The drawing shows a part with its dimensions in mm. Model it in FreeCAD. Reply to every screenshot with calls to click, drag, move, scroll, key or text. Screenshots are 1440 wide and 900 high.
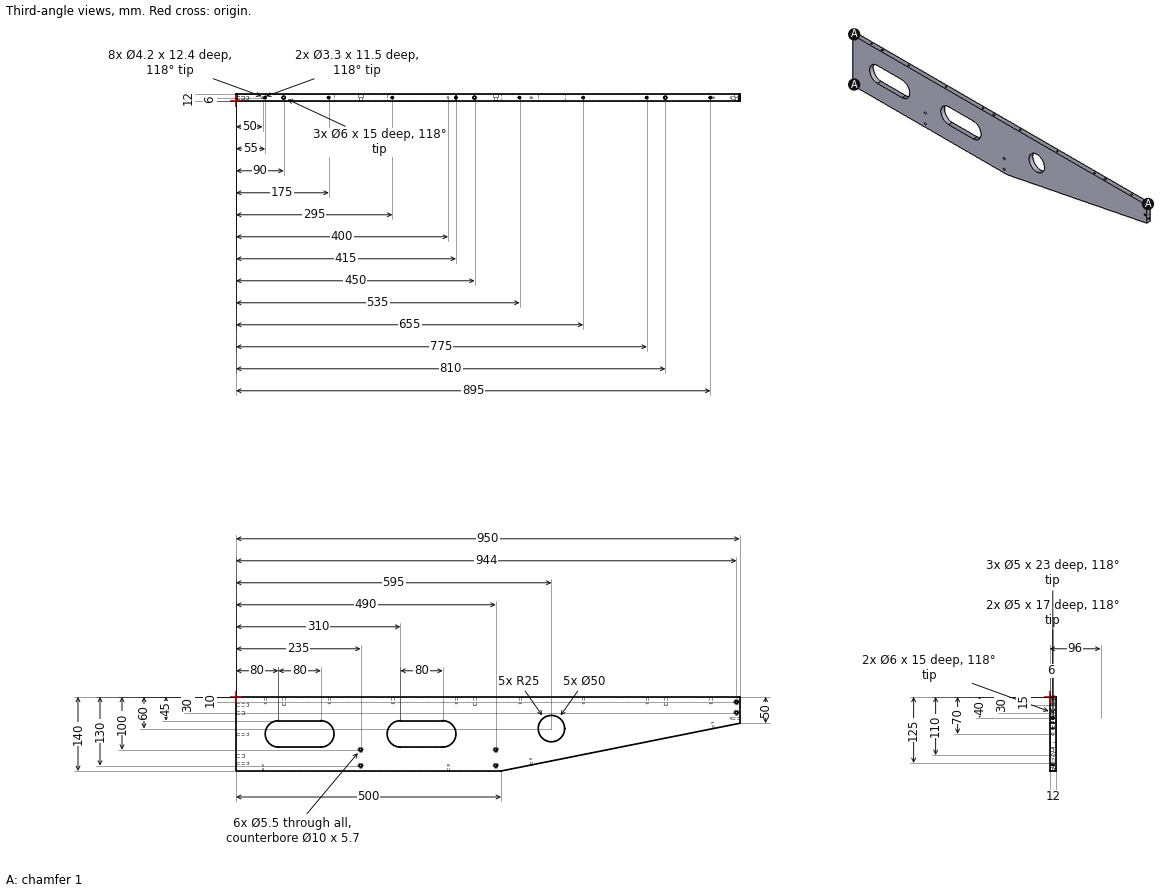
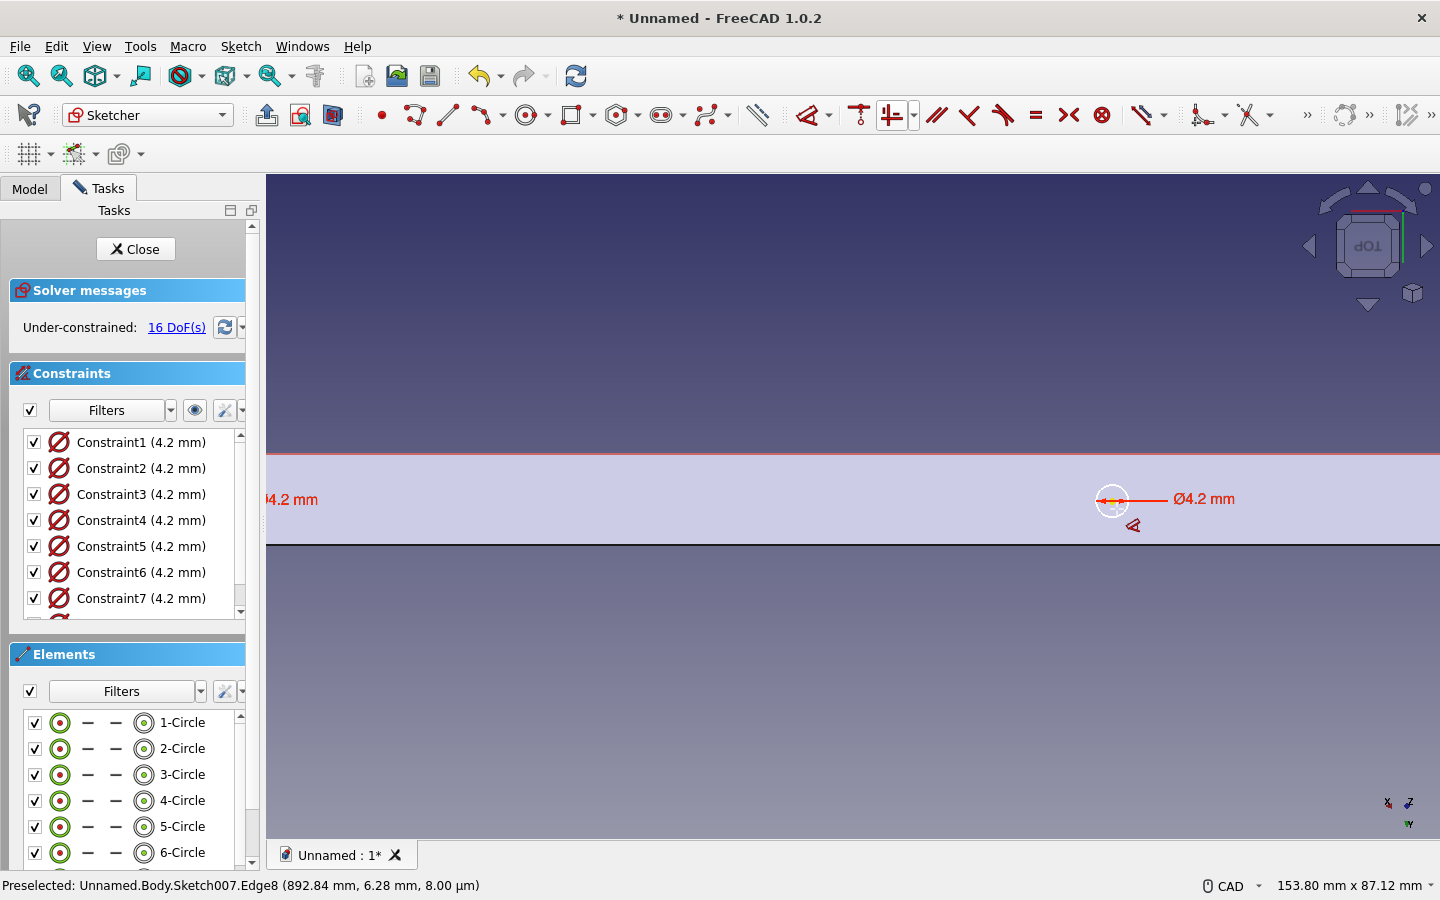
click(1112, 501)
click(1078, 478)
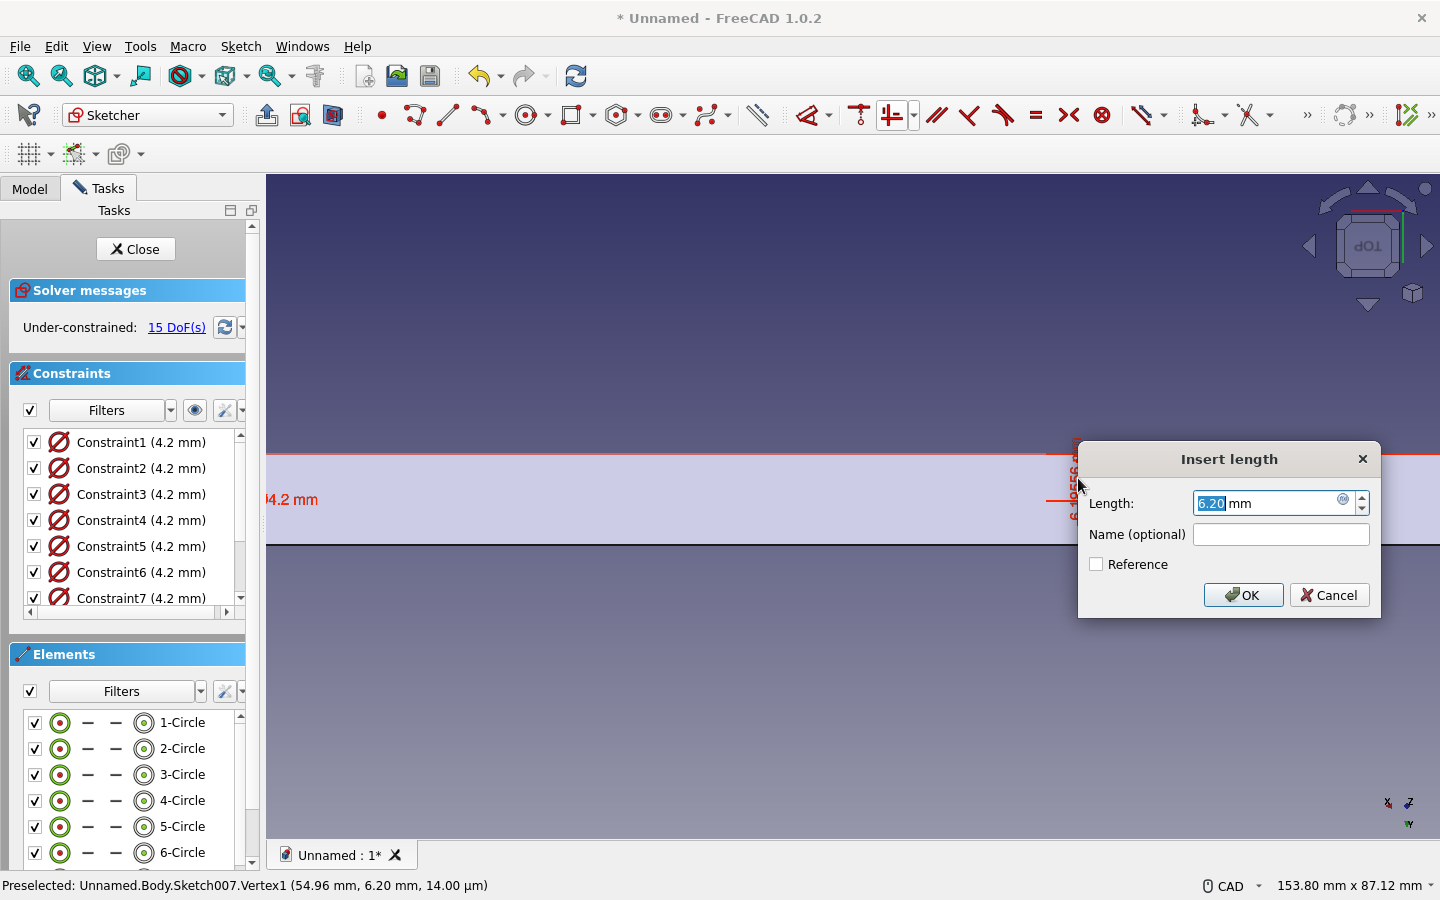
text(6)
key(Return)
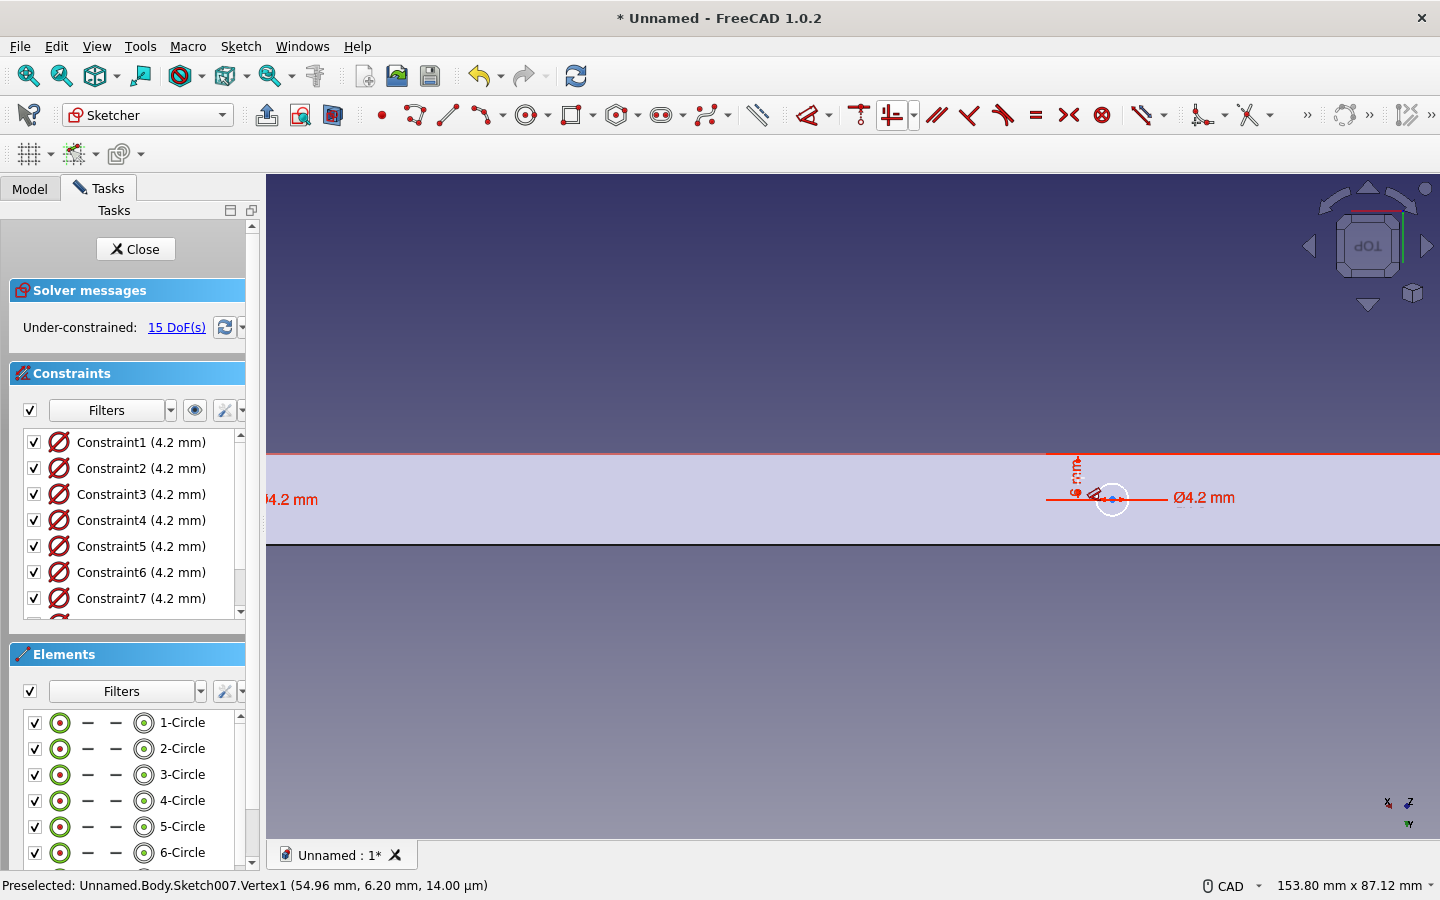
scroll(1118, 509, down, 11)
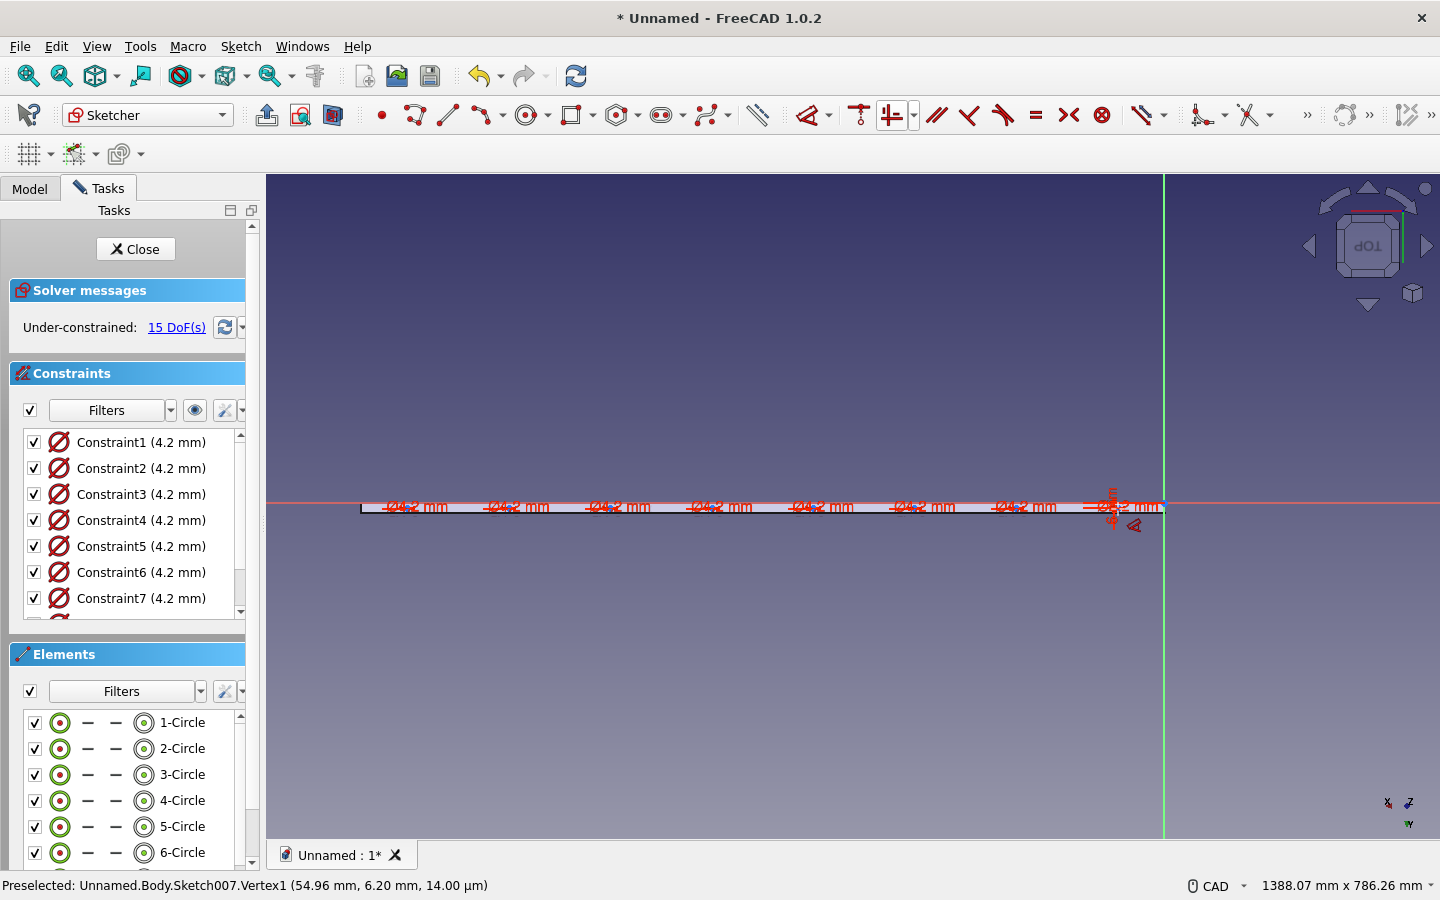
scroll(1016, 509, up, 11)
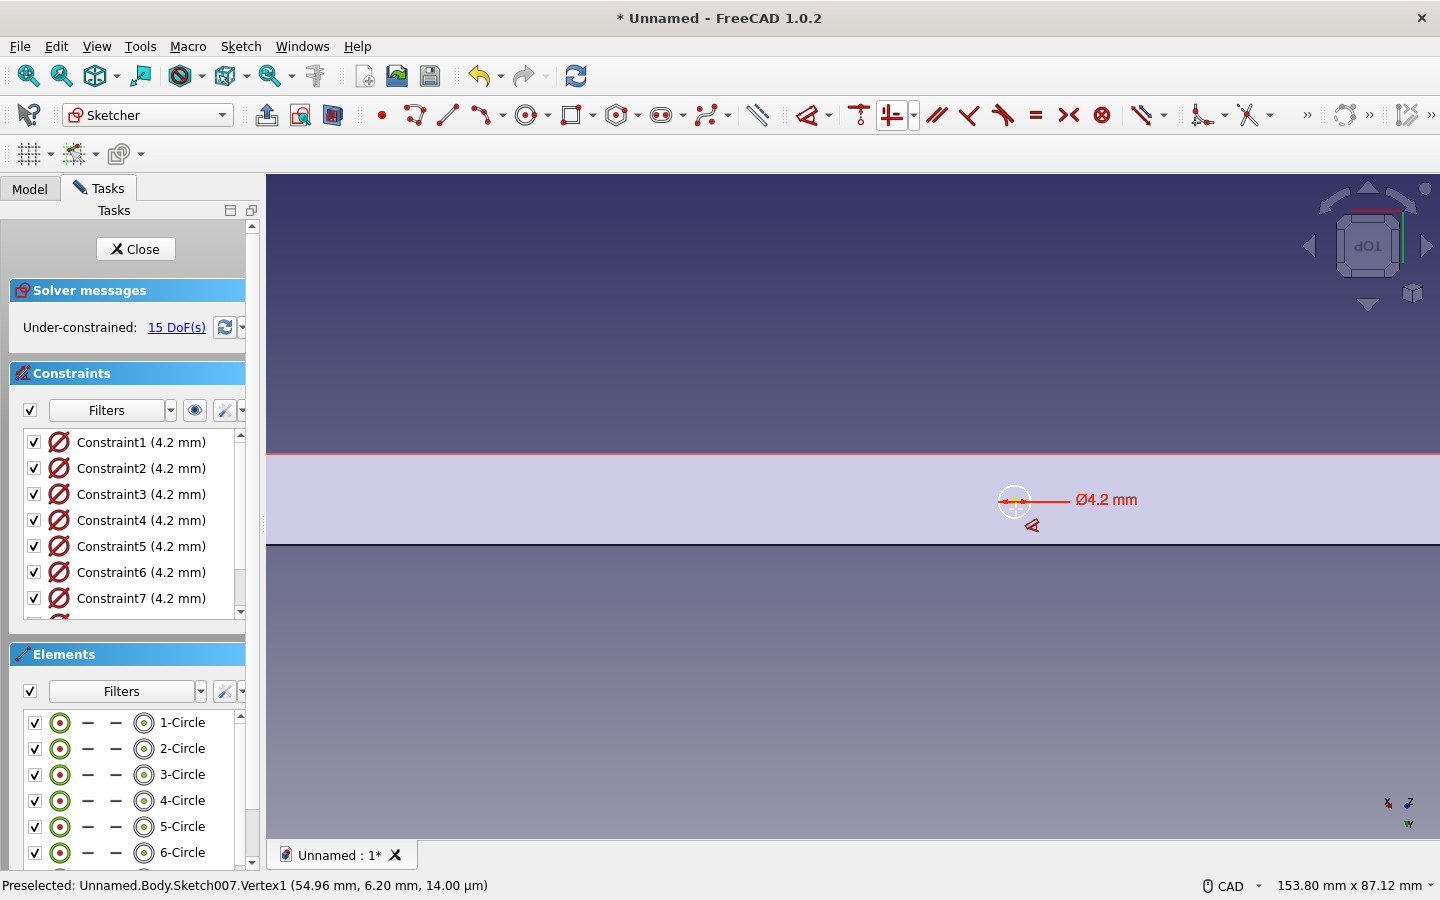
click(1015, 502)
click(981, 478)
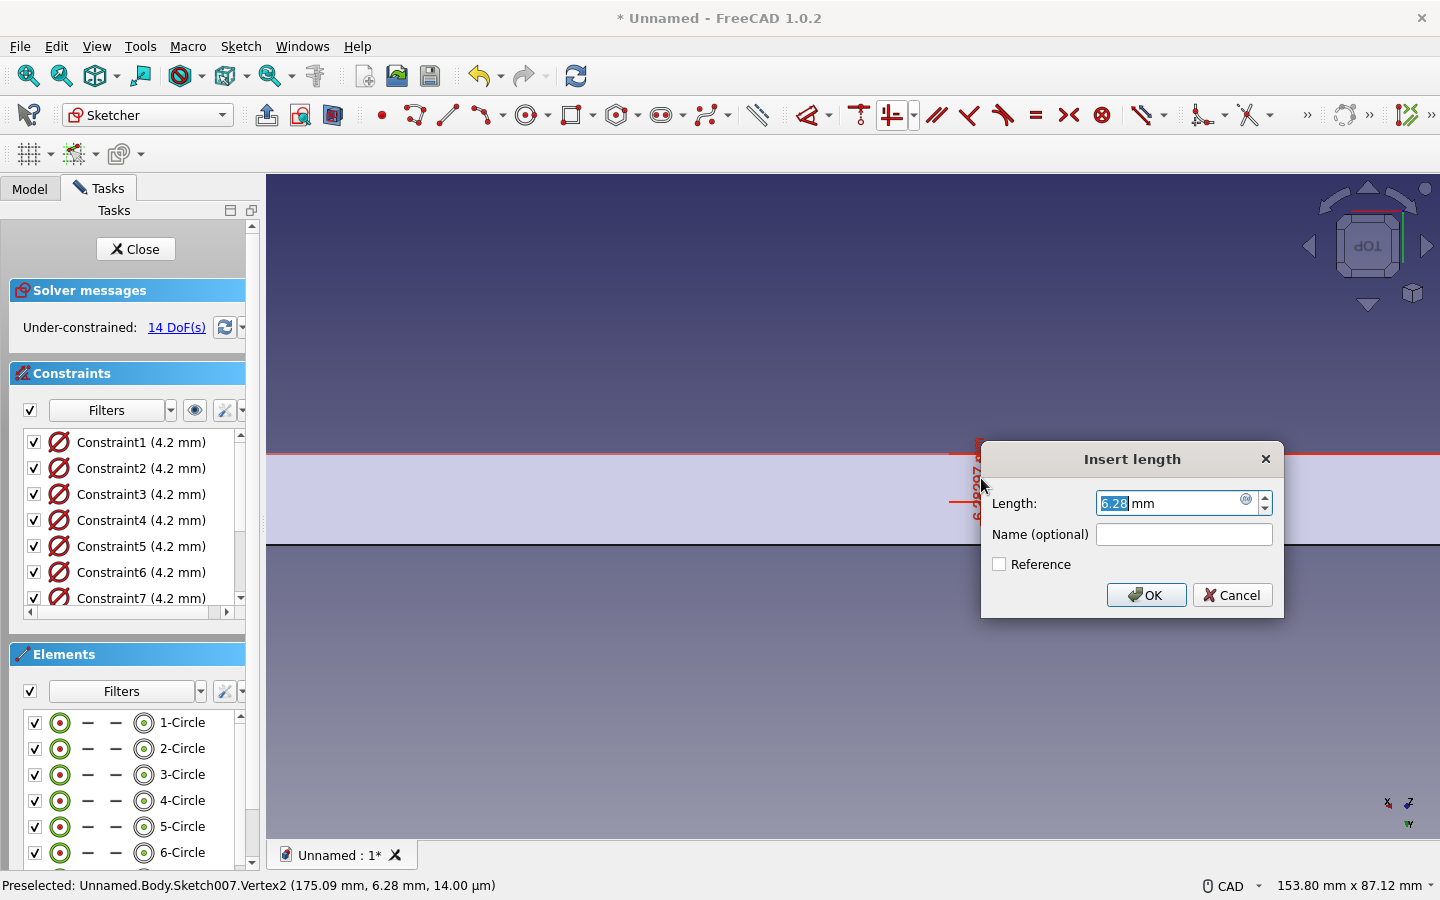
text(6)
key(Return)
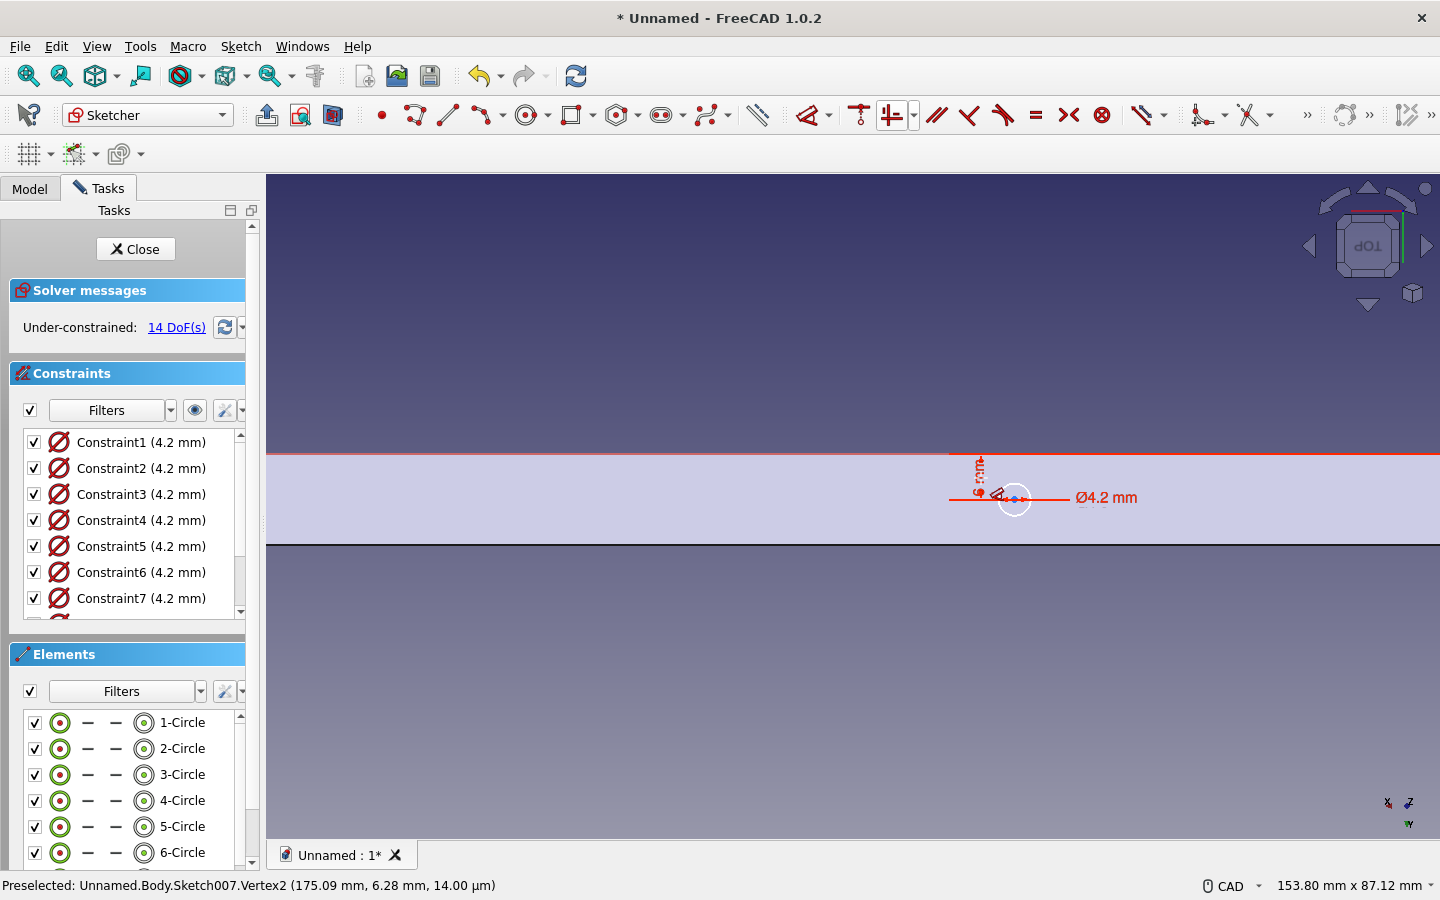
scroll(1016, 509, down, 11)